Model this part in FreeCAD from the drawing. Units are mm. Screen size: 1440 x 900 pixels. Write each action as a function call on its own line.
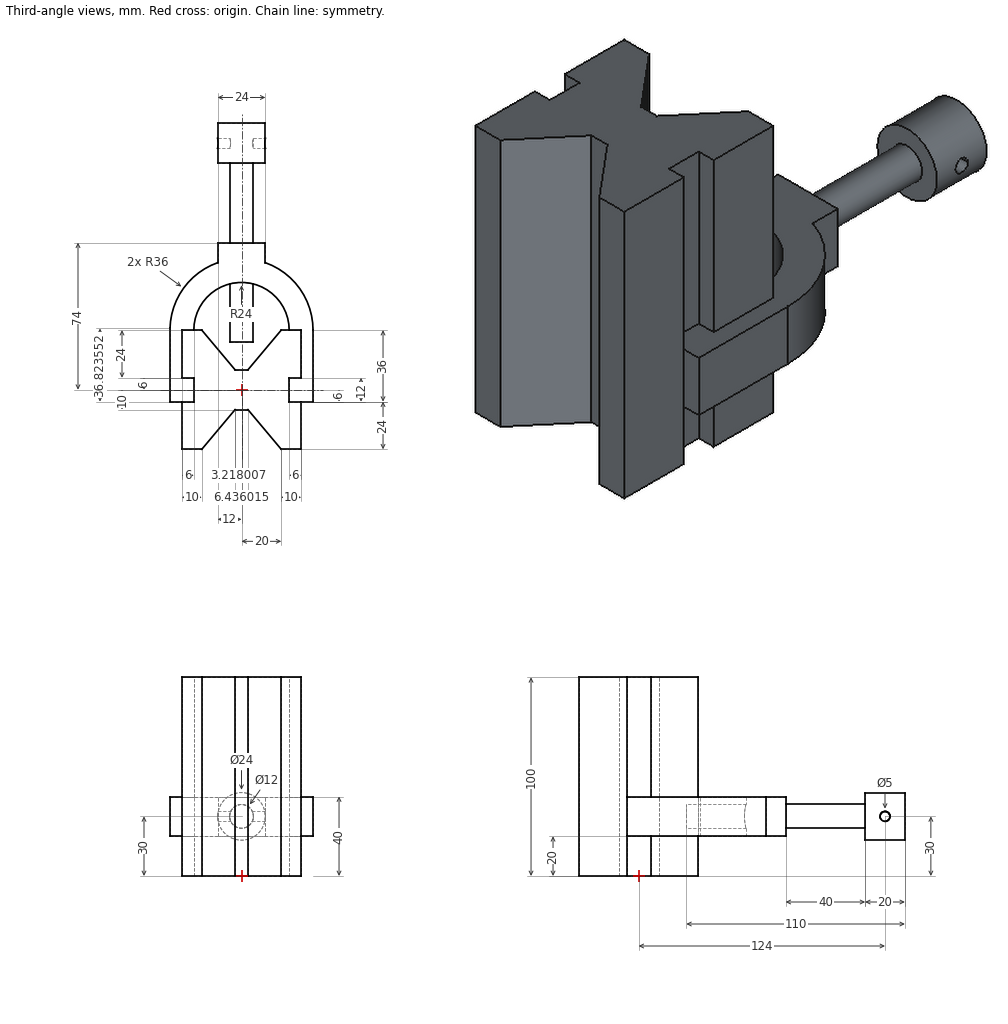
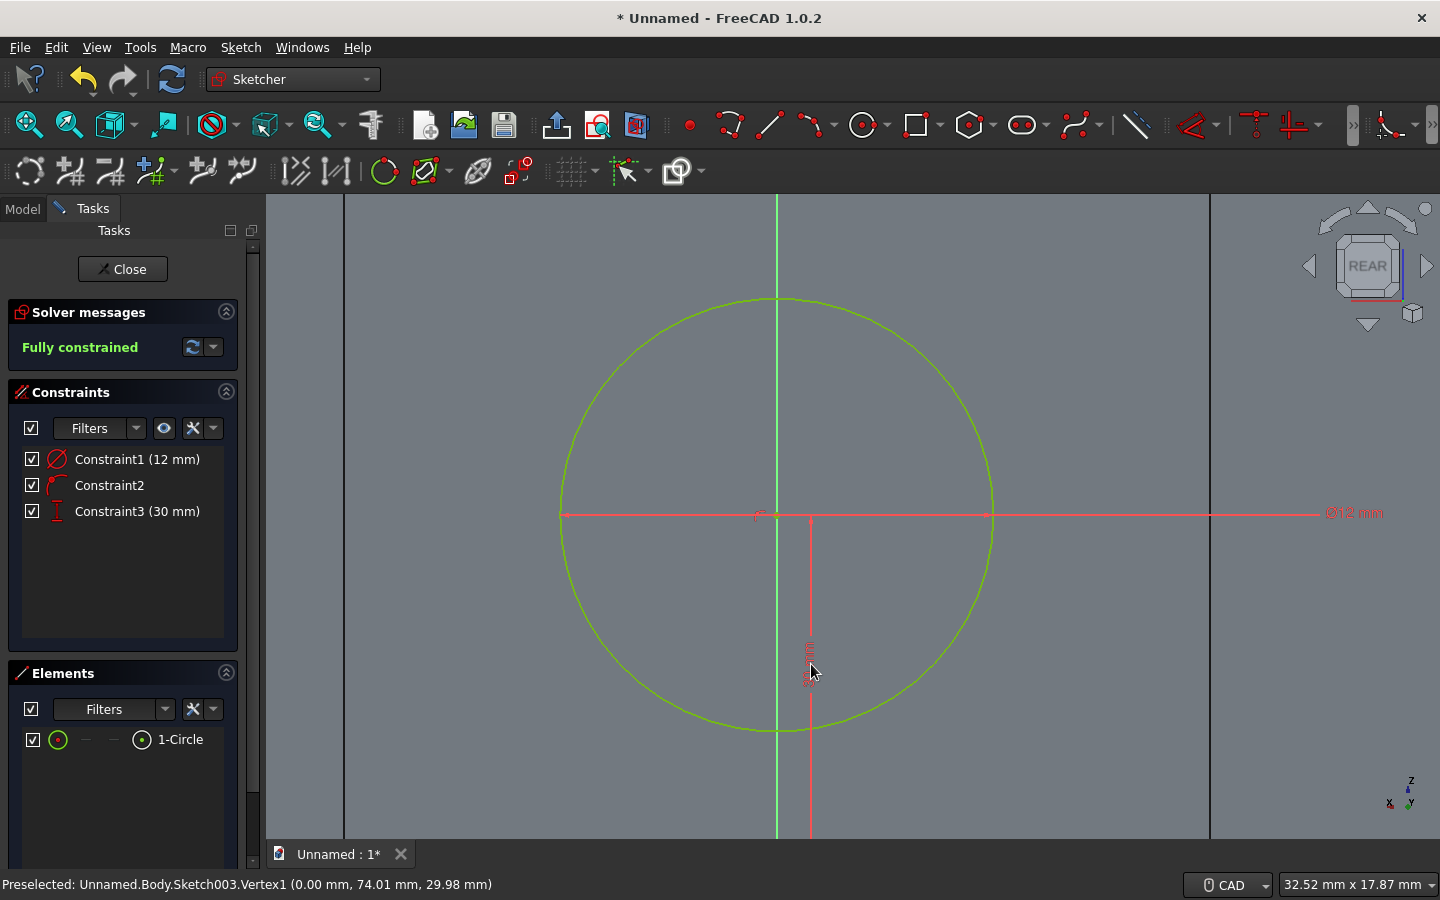
click(123, 269)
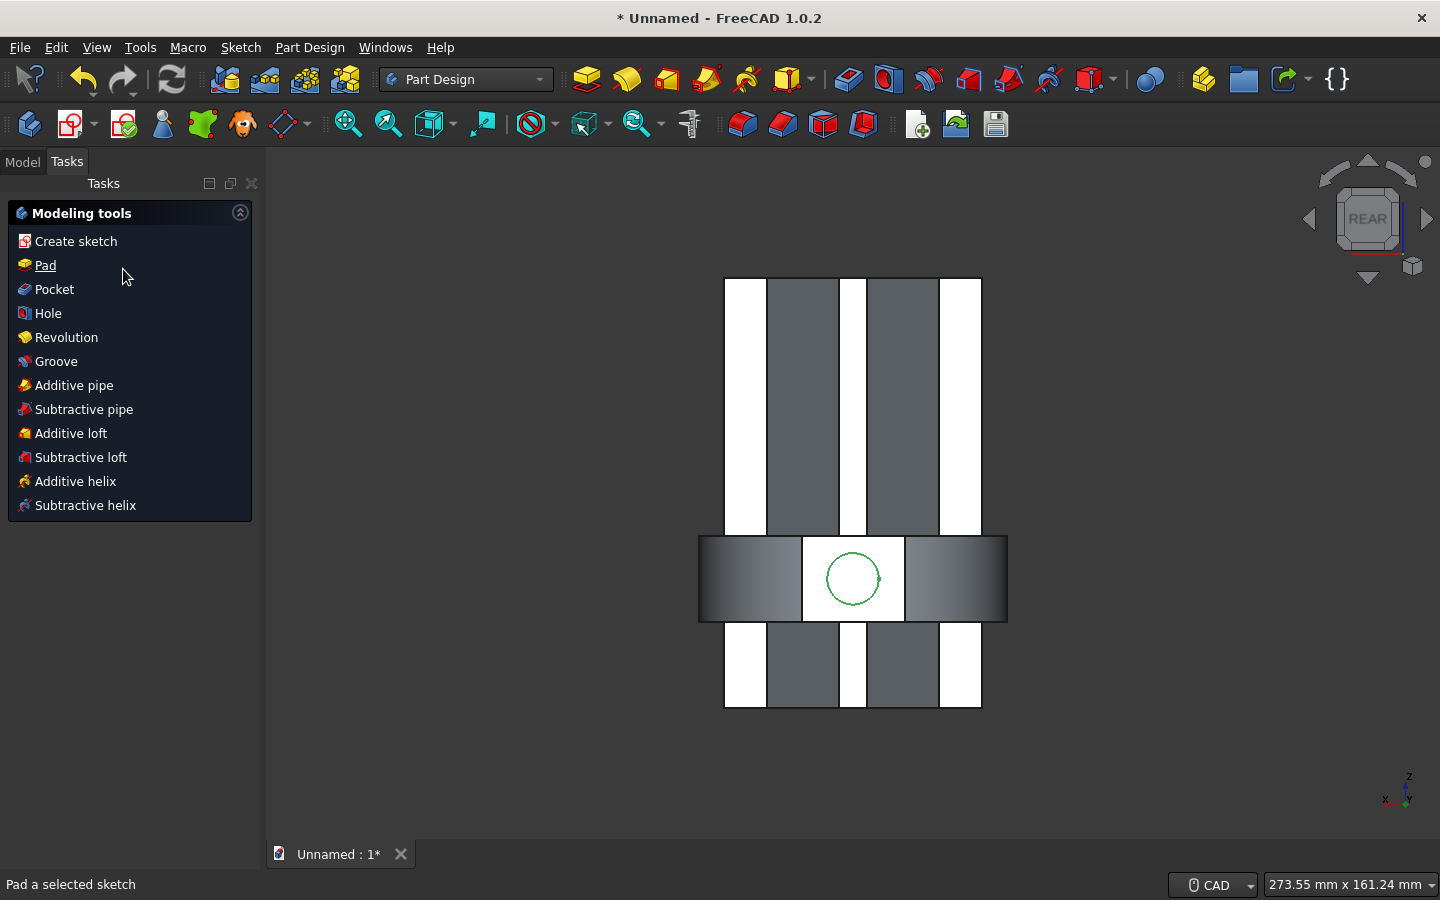
click(588, 80)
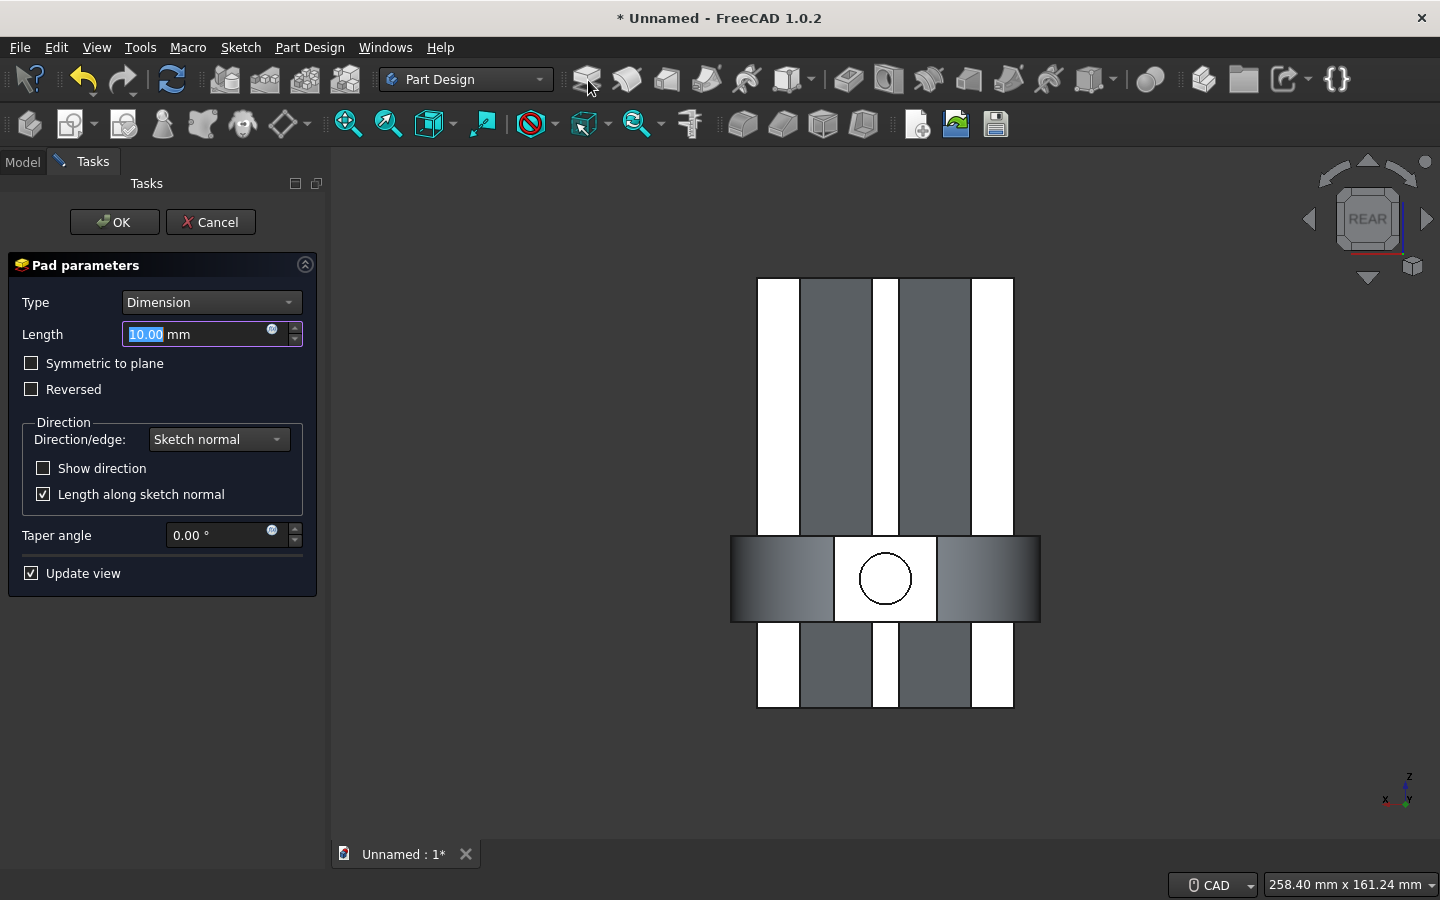
text(40)
key(Tab)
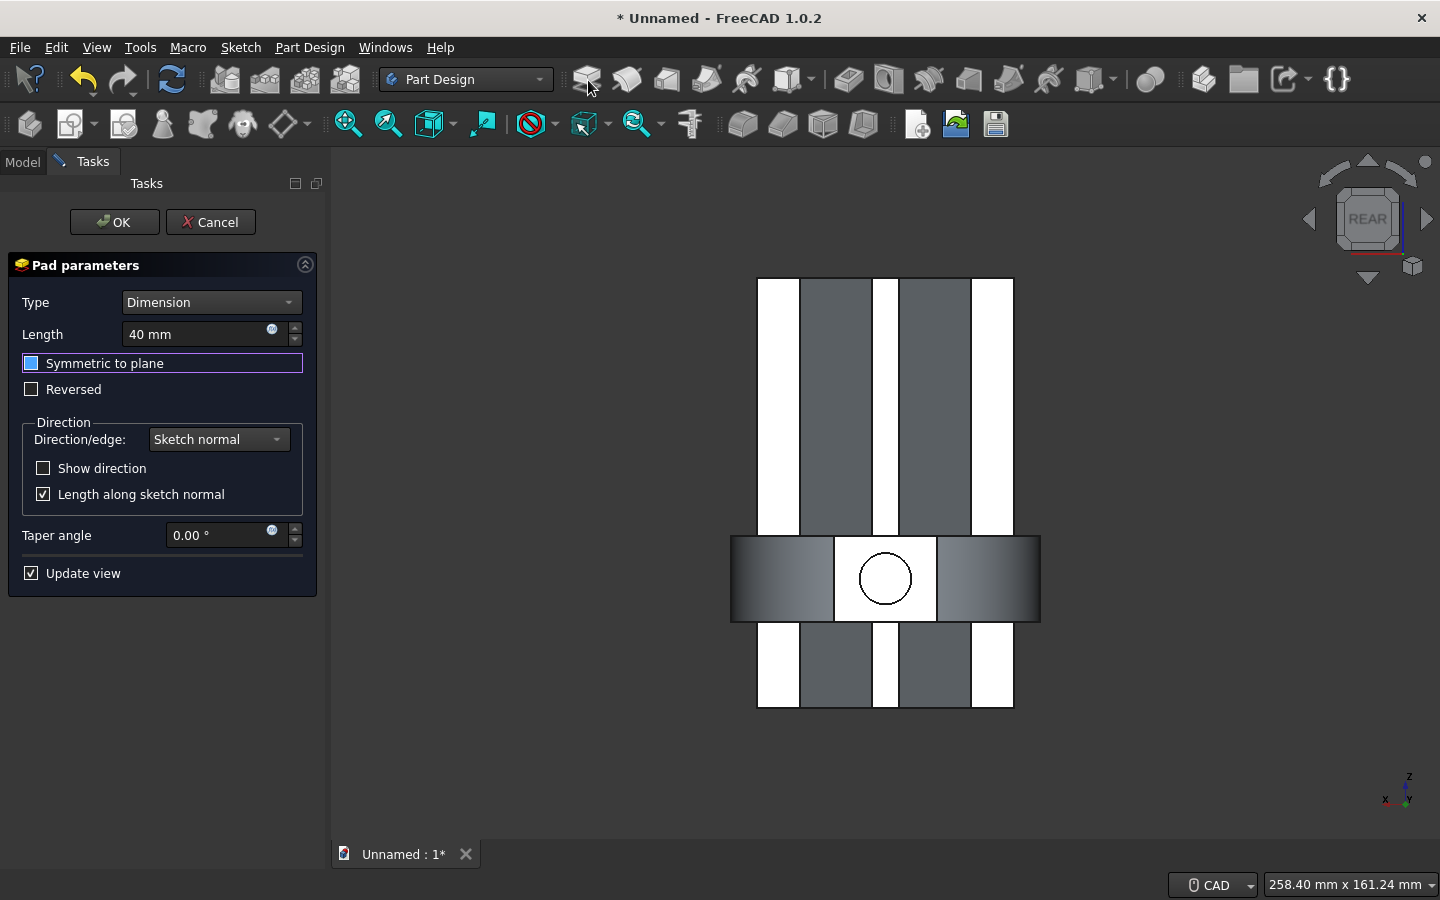
click(115, 222)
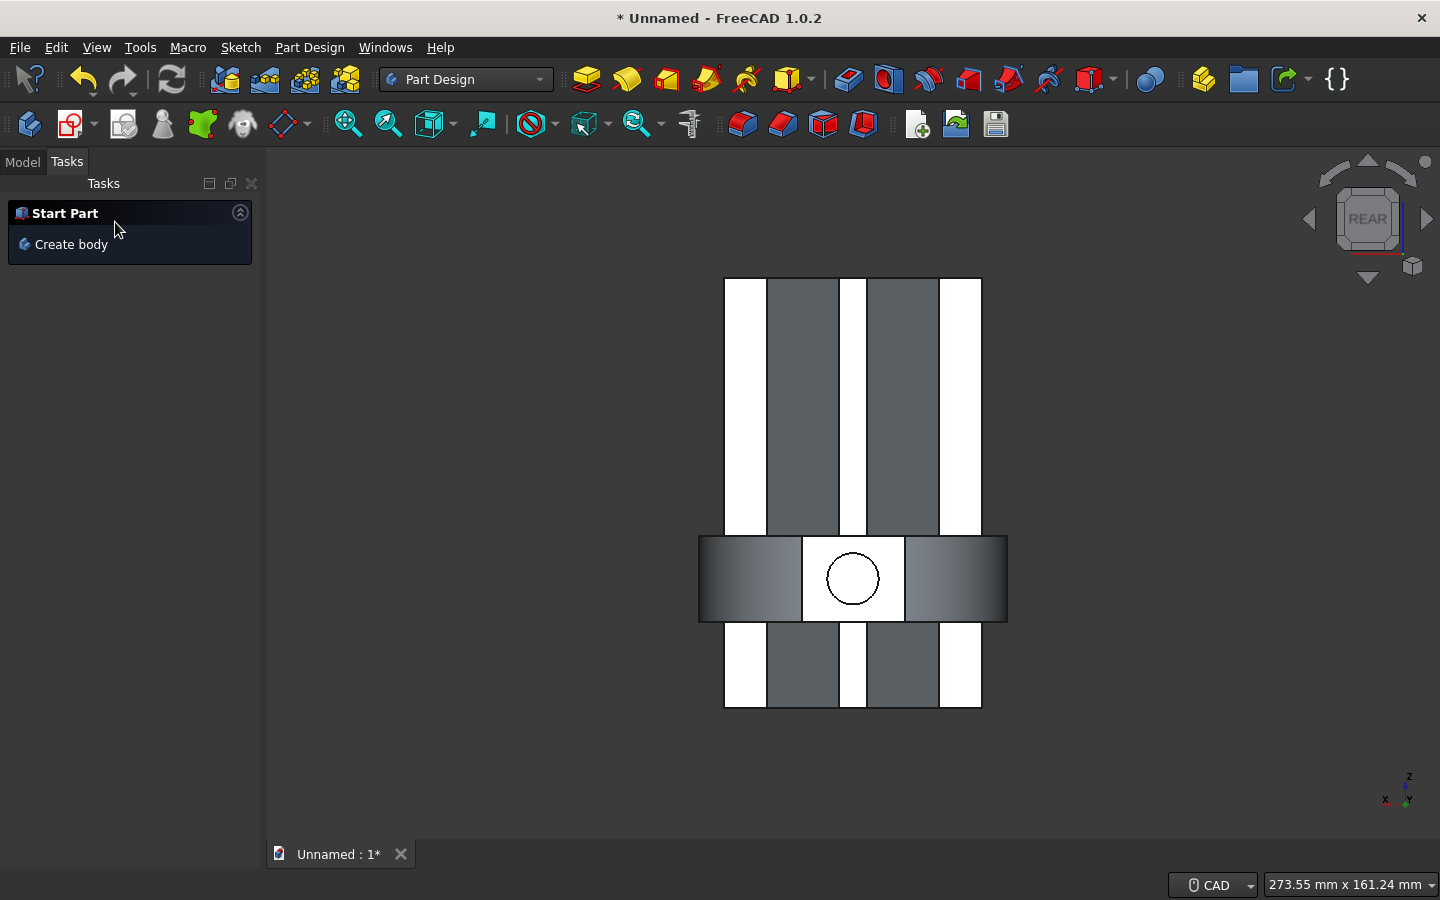
click(853, 578)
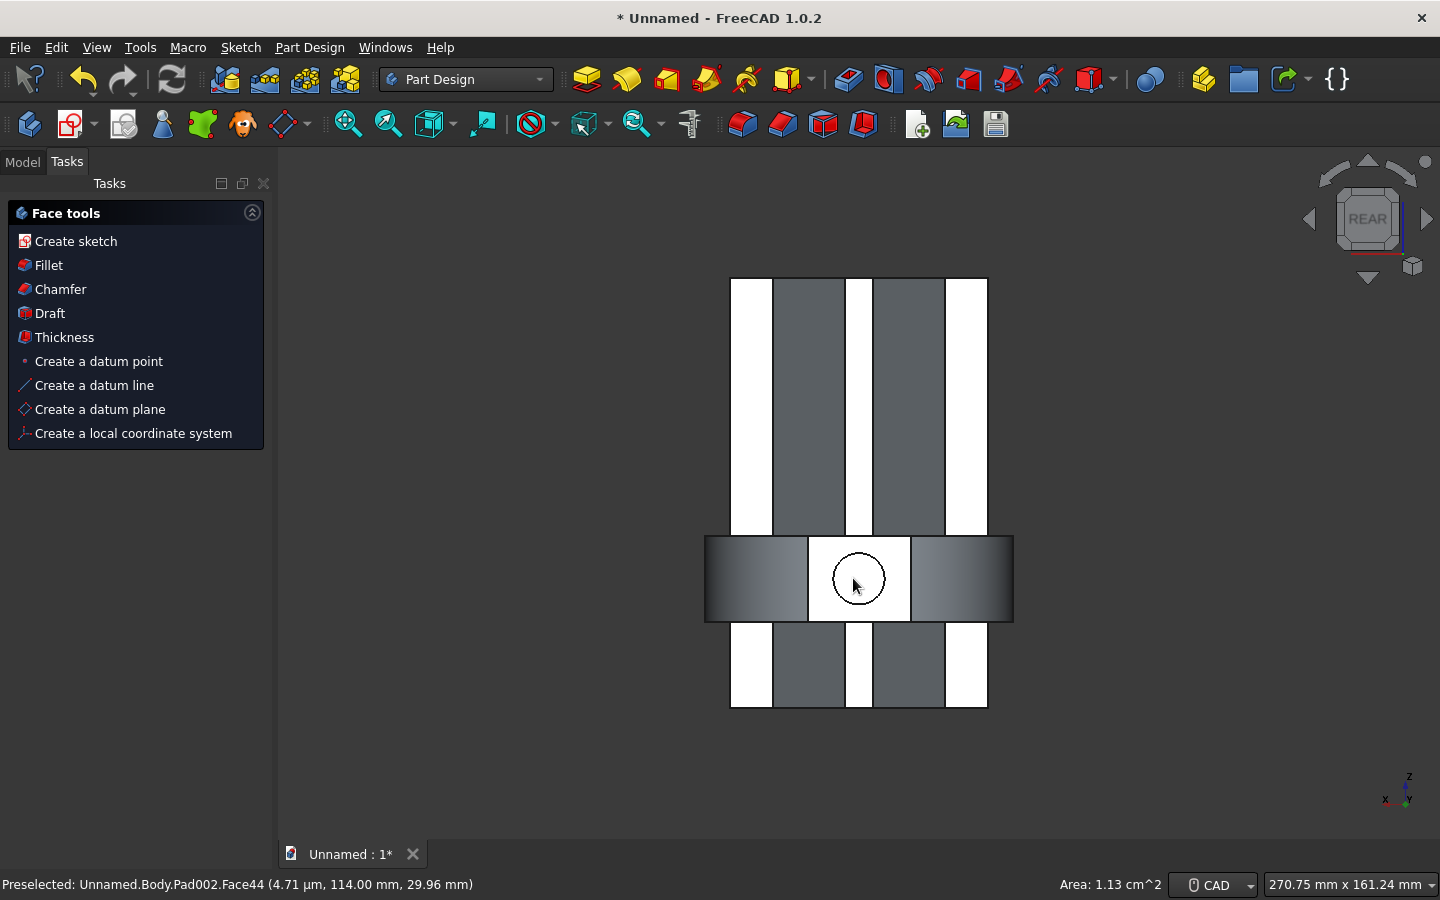
click(70, 124)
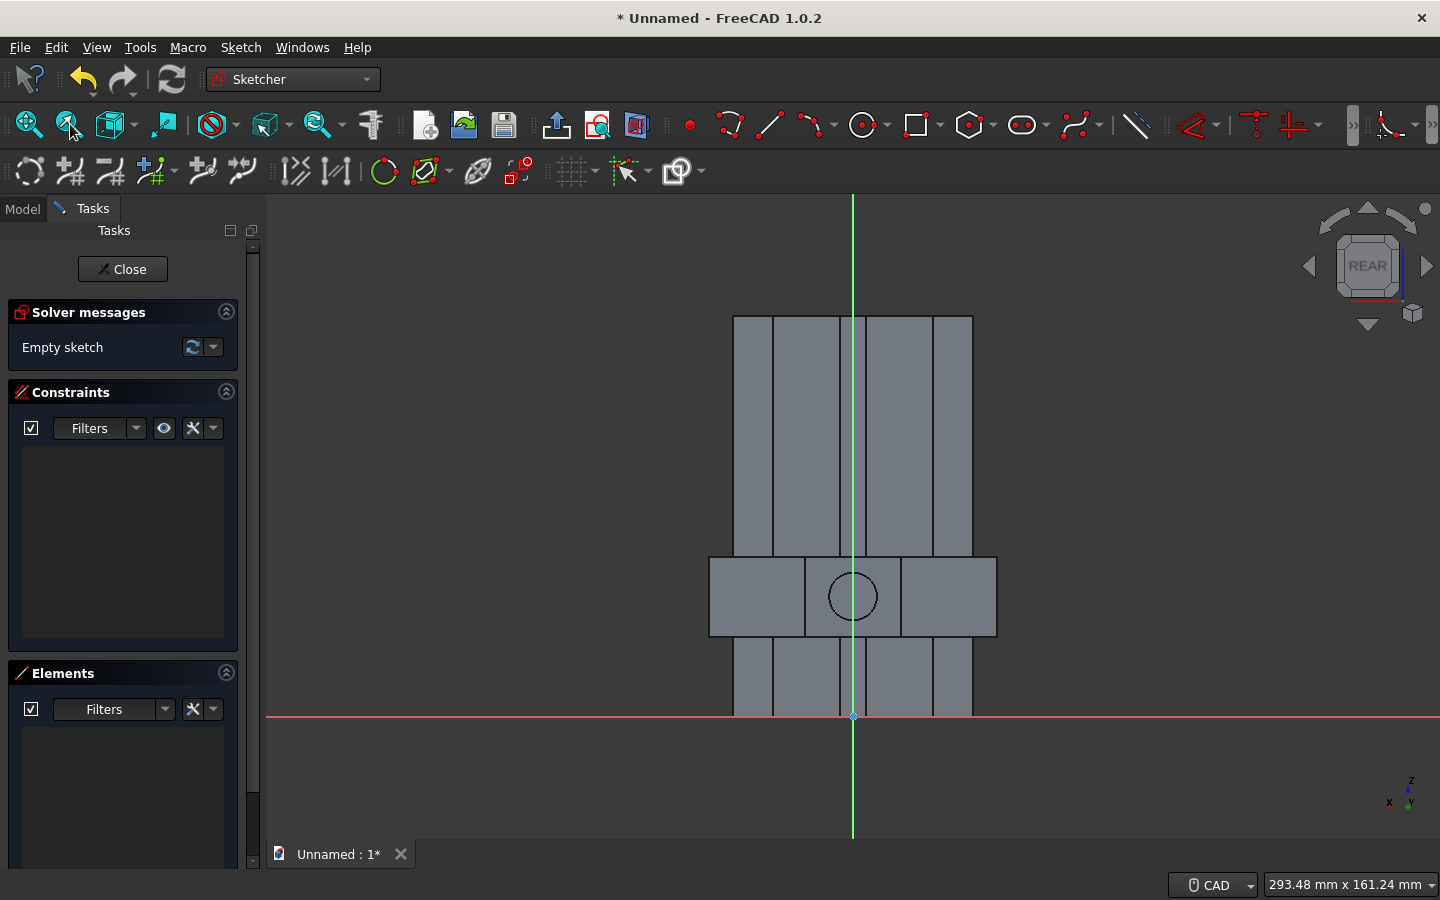
scroll(893, 700, up, 5)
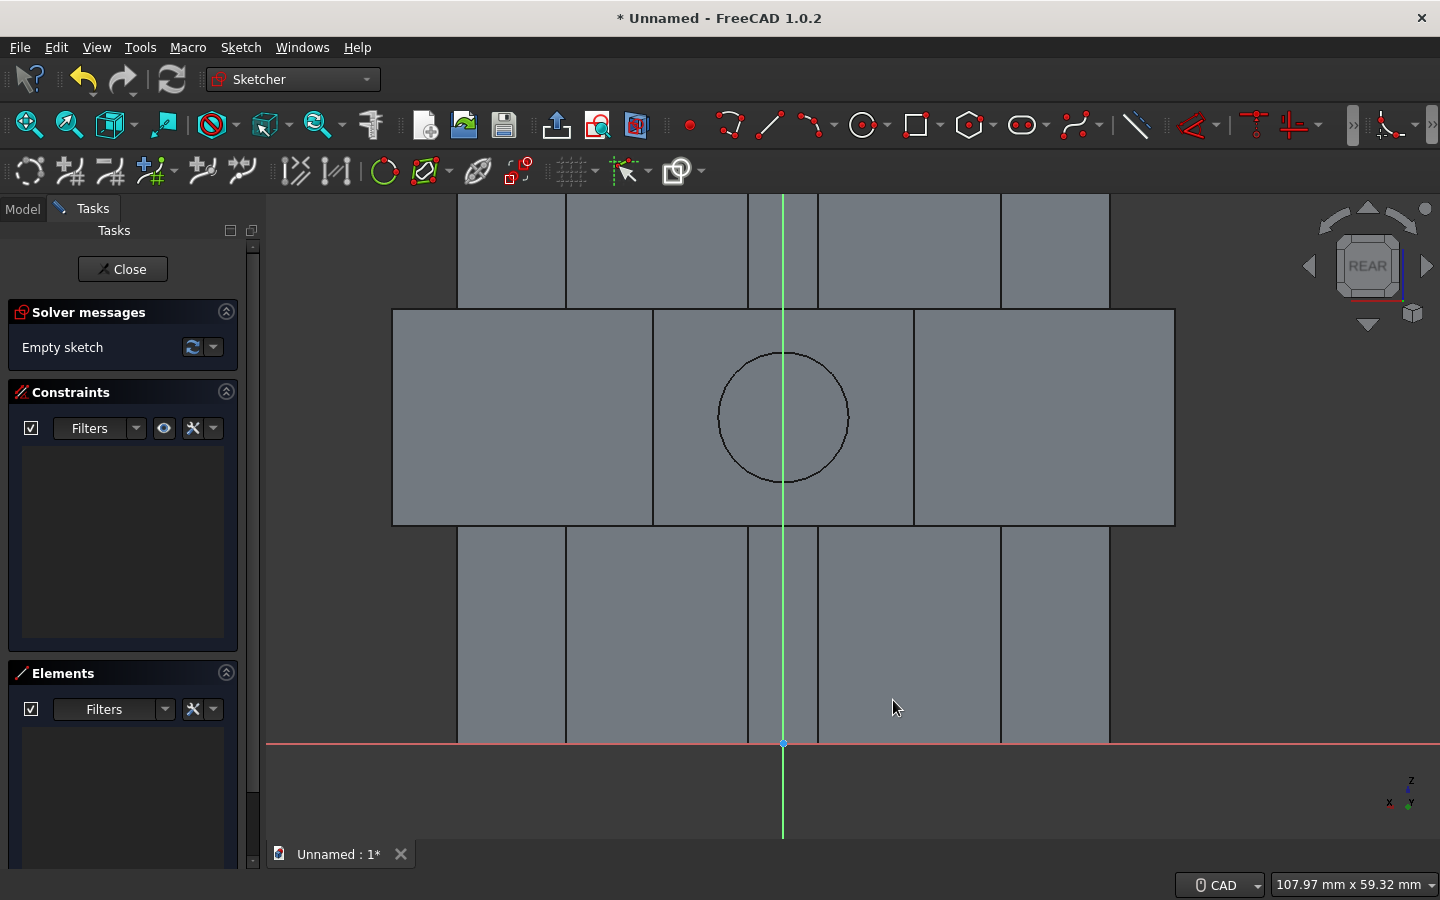
key(g)
key(c)